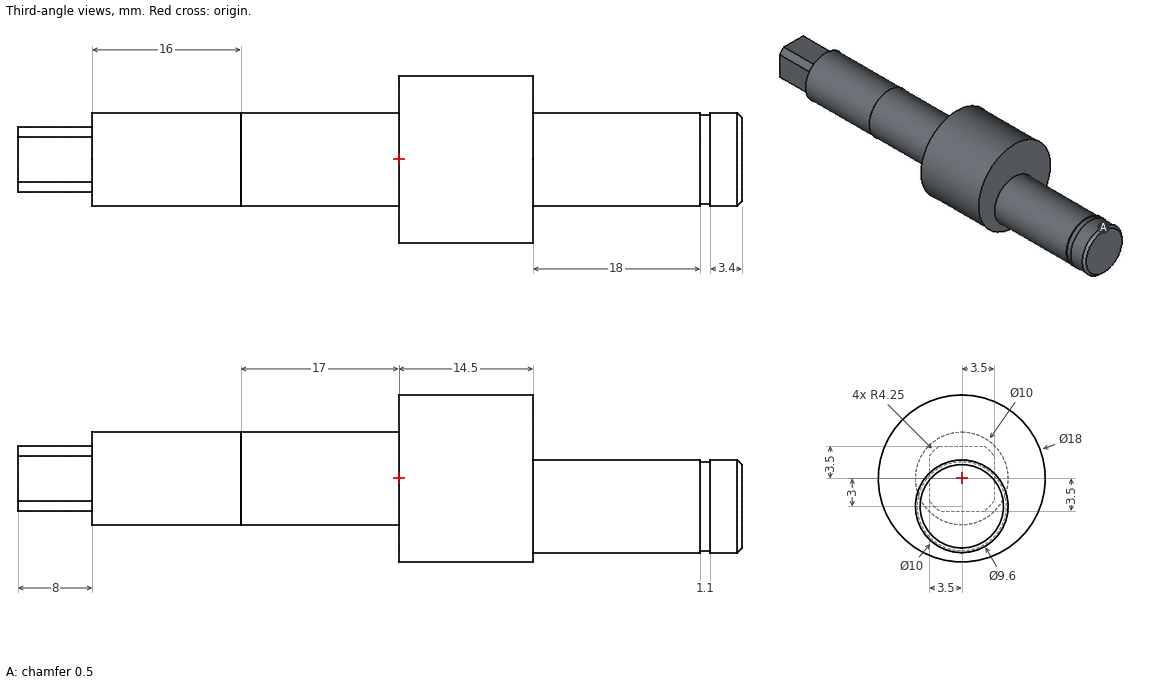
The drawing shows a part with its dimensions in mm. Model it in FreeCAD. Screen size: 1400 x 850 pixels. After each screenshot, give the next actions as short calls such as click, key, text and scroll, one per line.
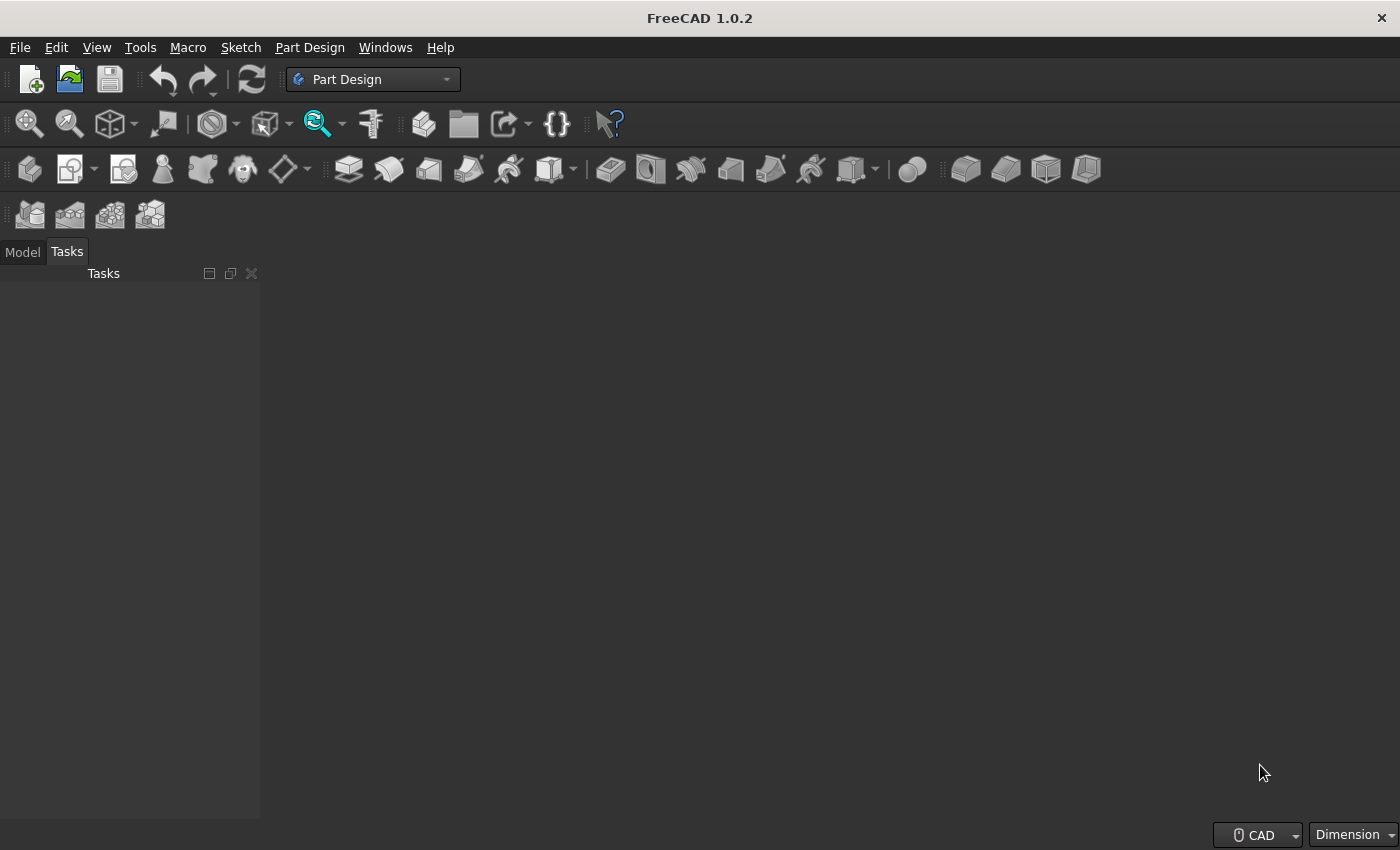
click(30, 80)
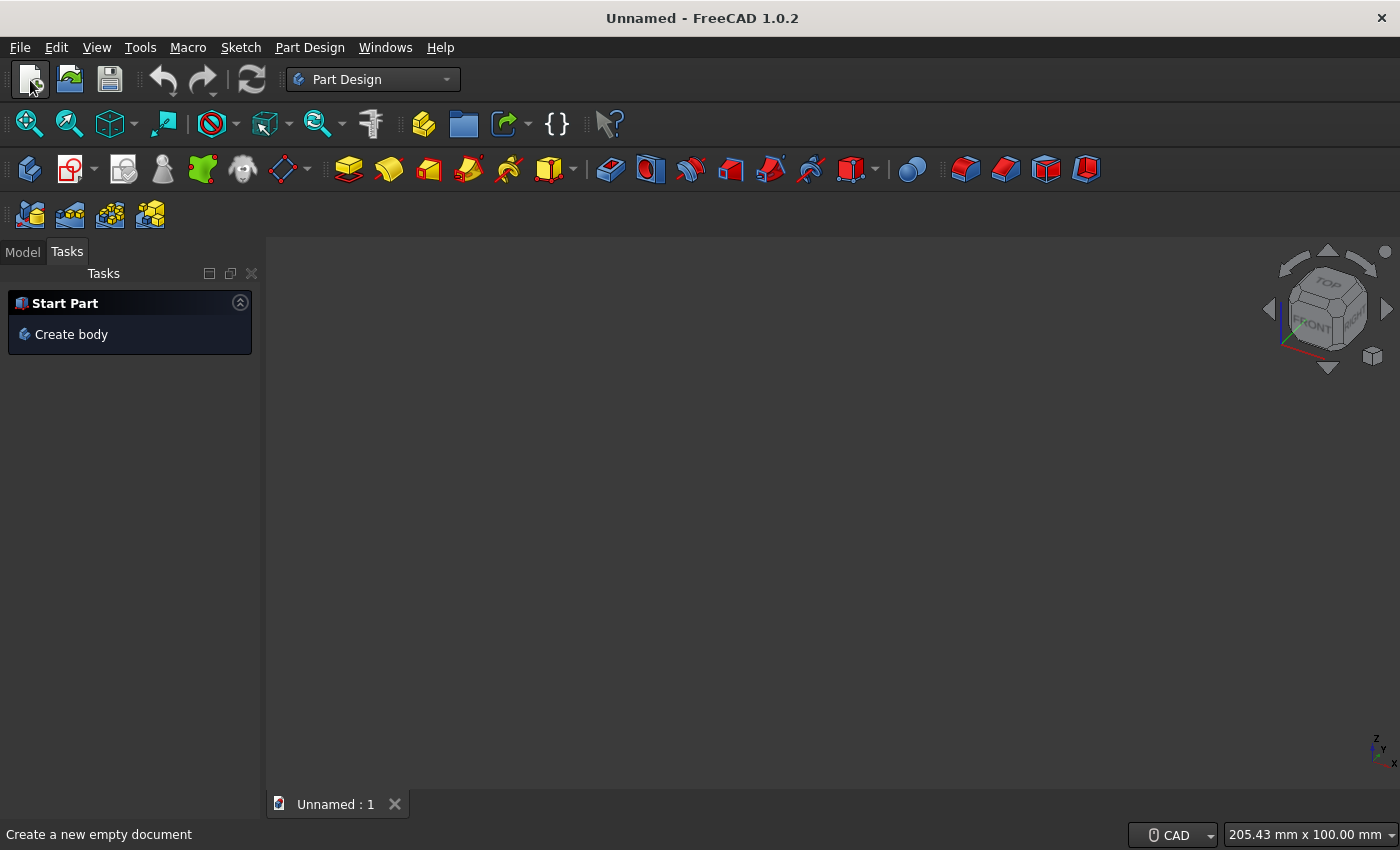
click(70, 170)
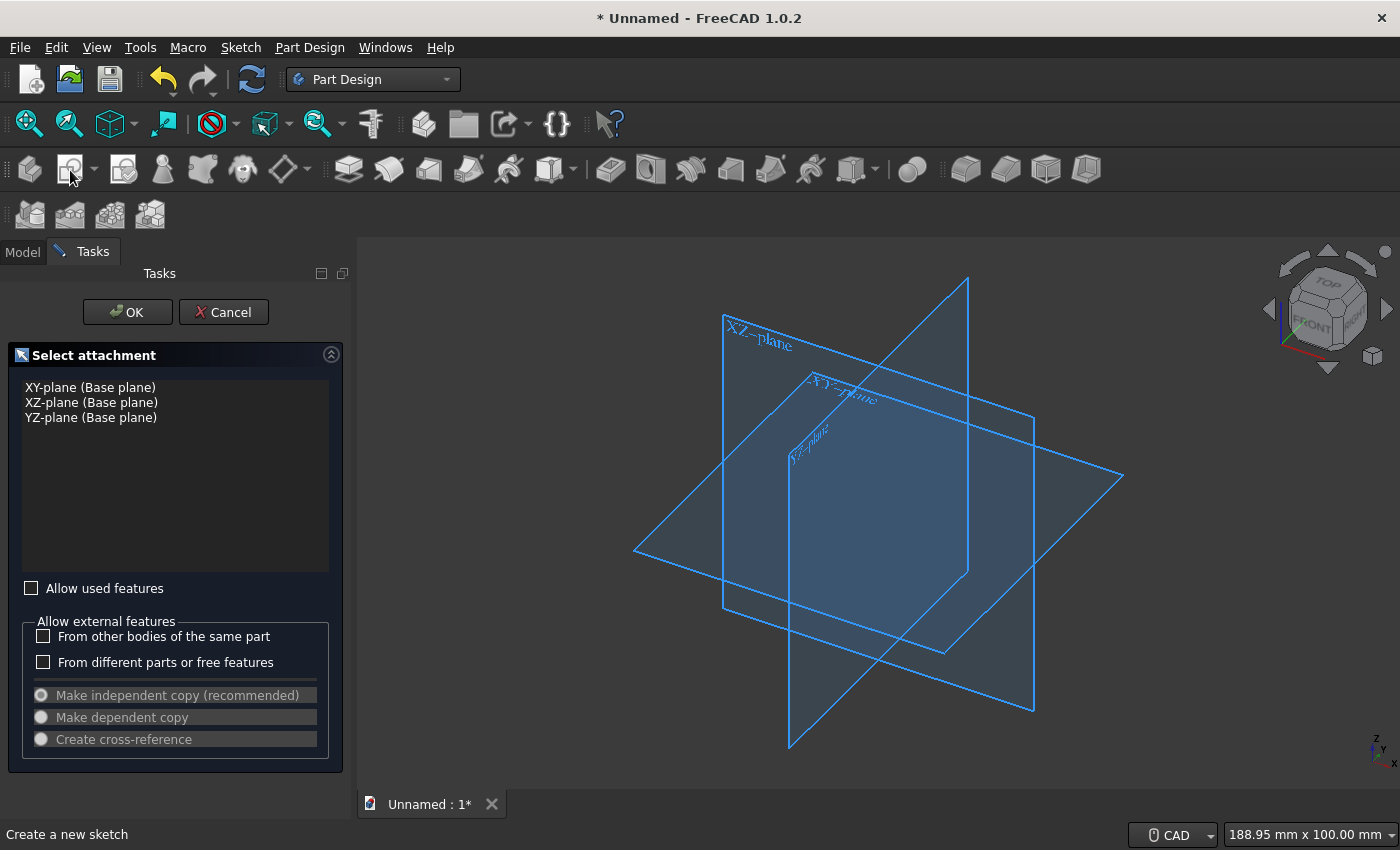
click(82, 418)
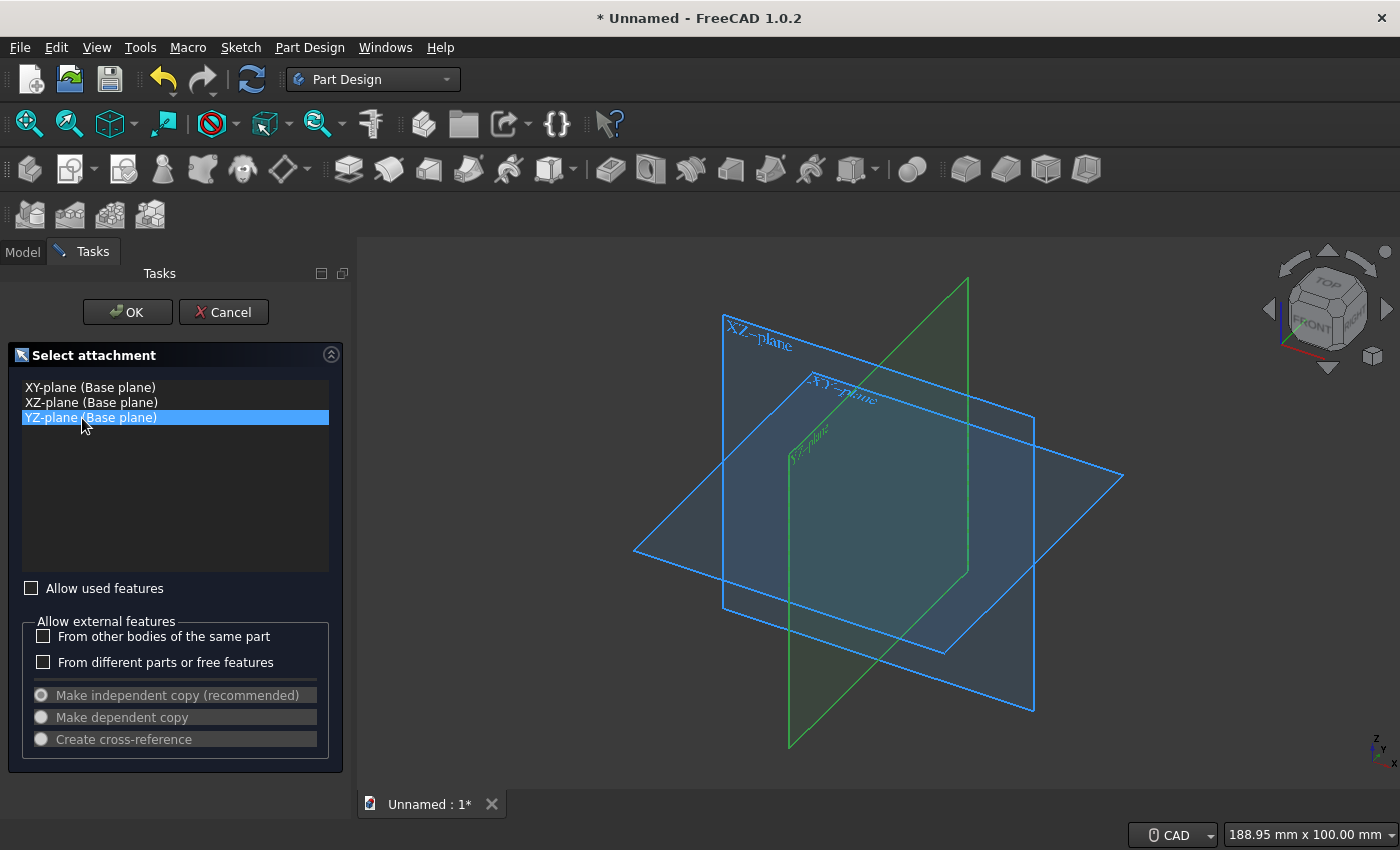
click(128, 312)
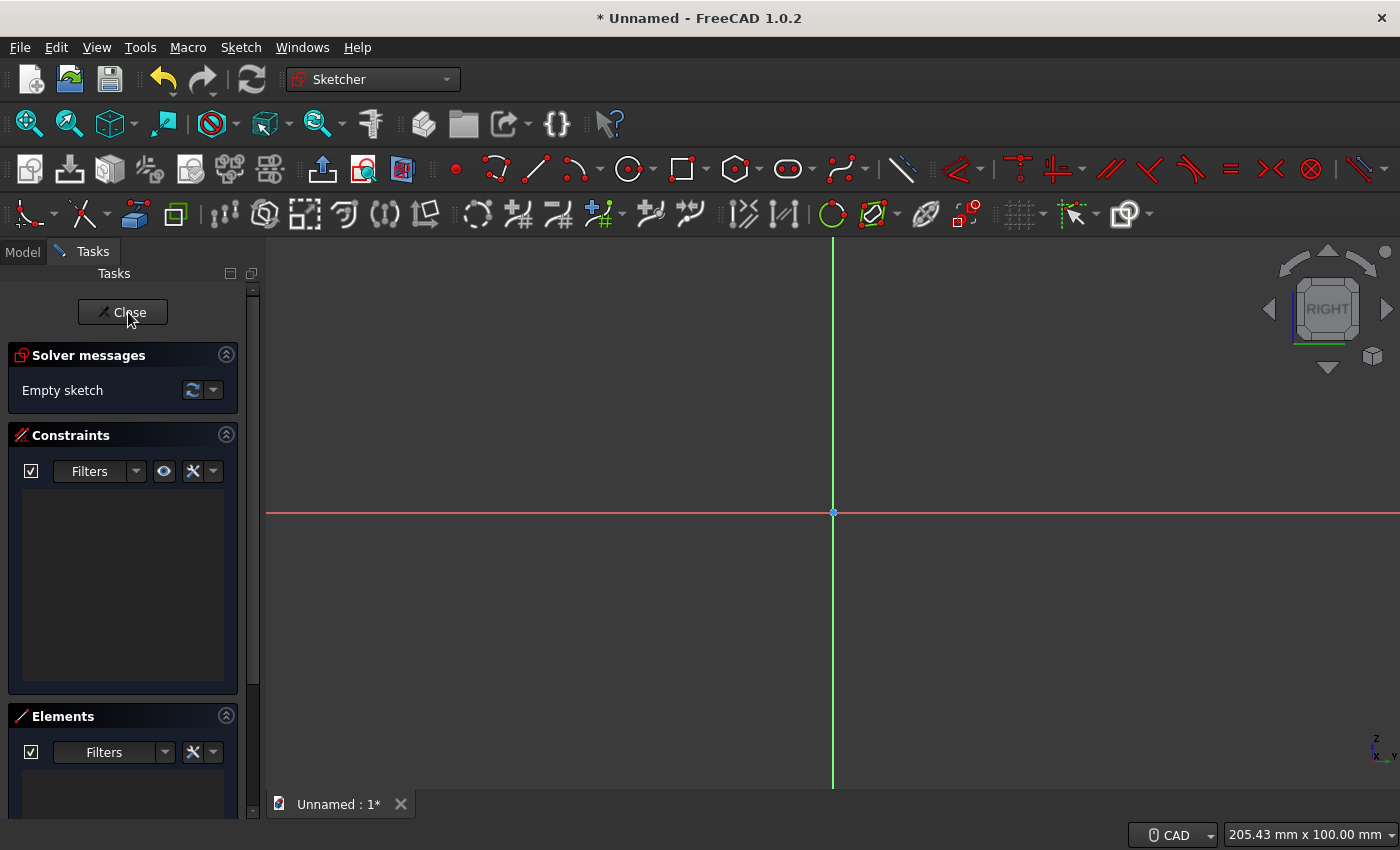
scroll(863, 513, up, 6)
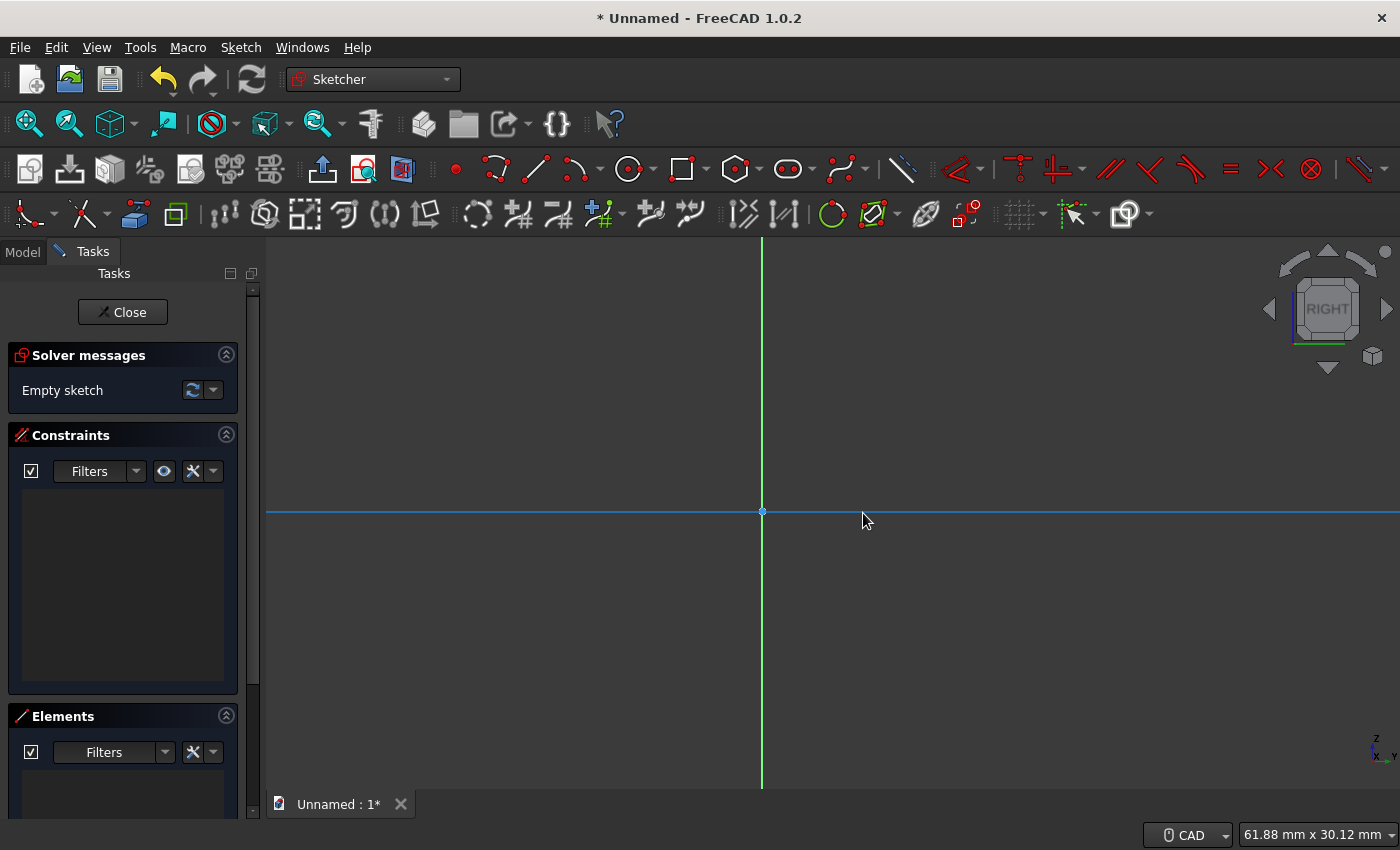
click(630, 170)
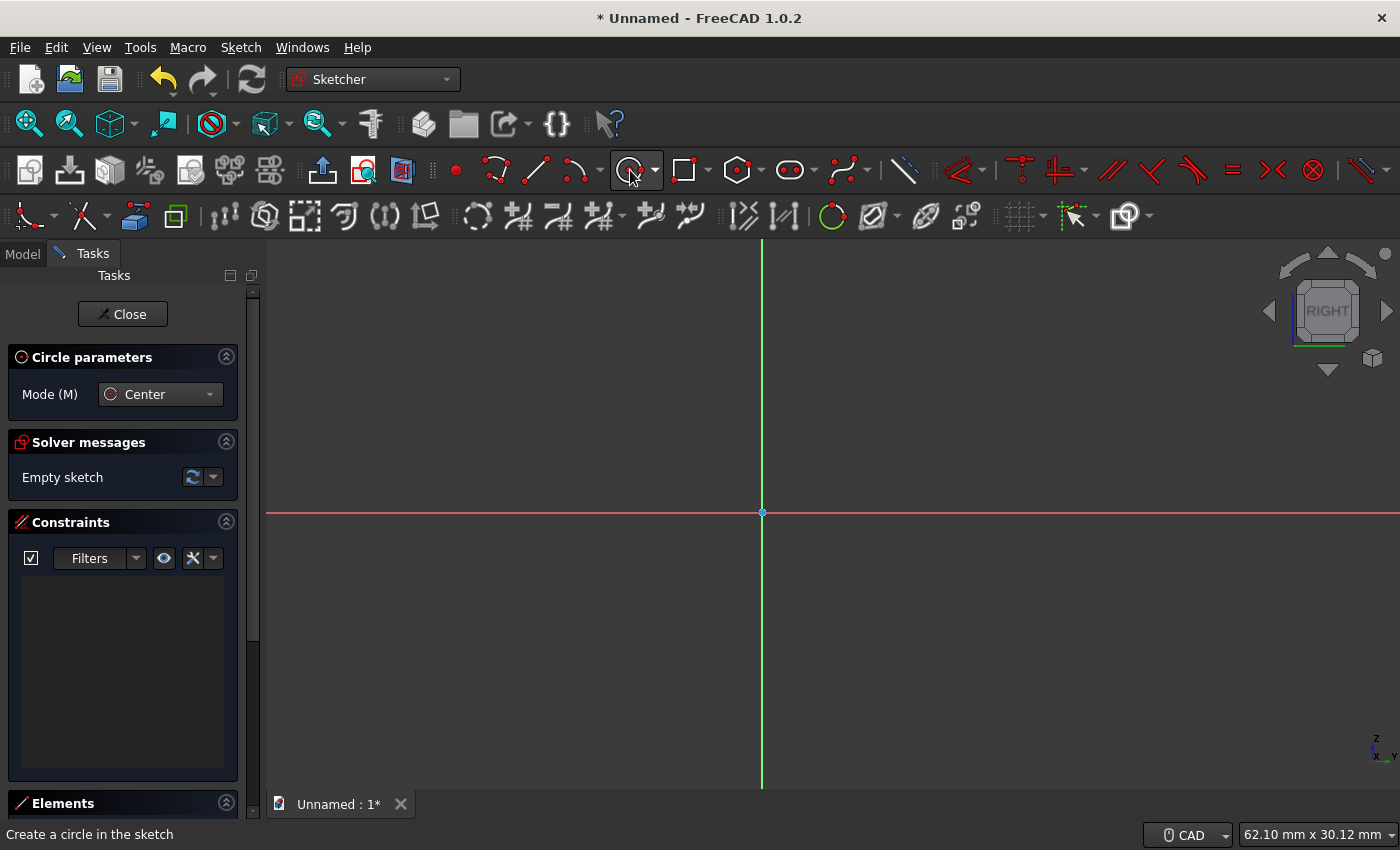
click(762, 513)
move(879, 397)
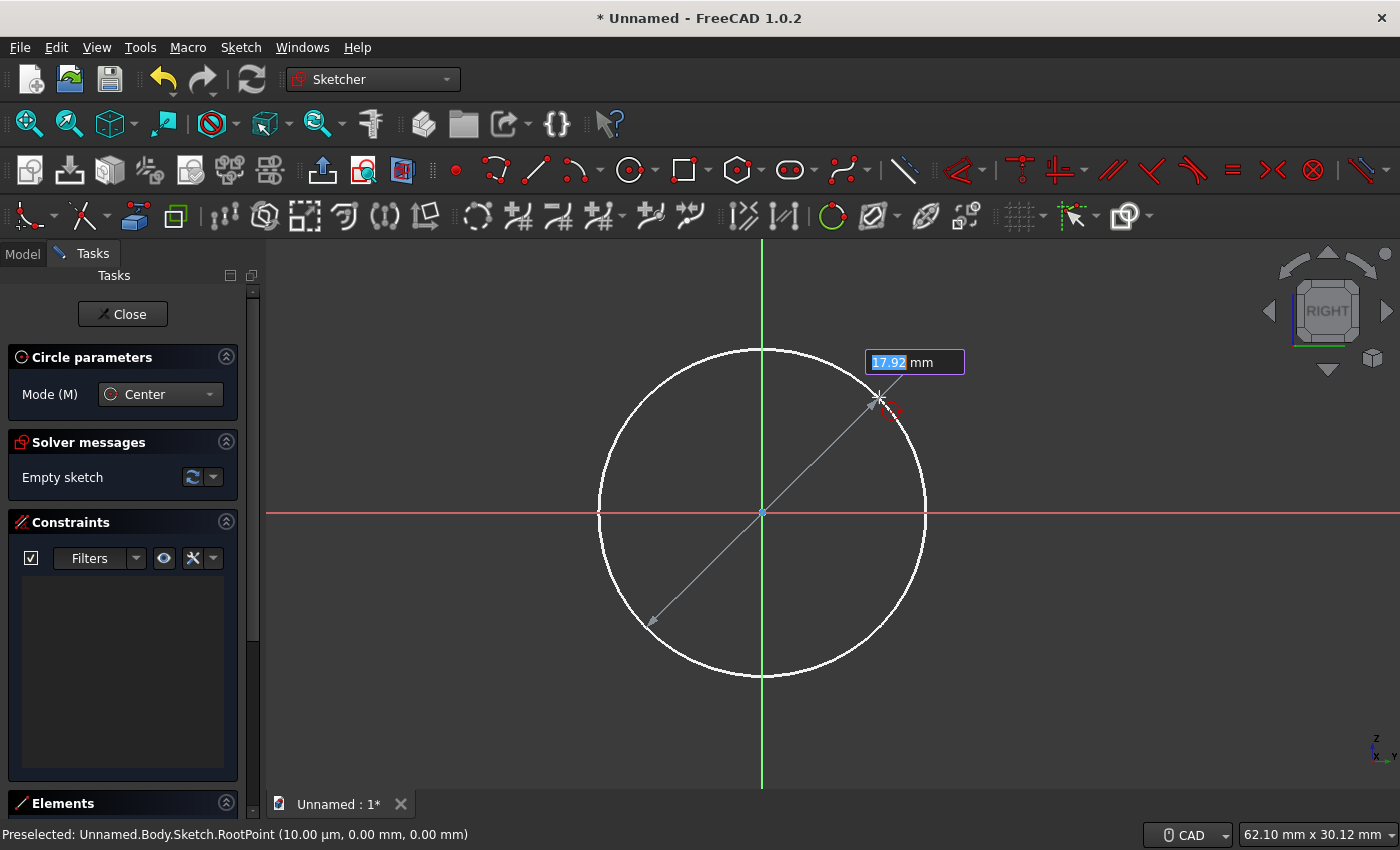
text(18)
key(Return)
key(Escape)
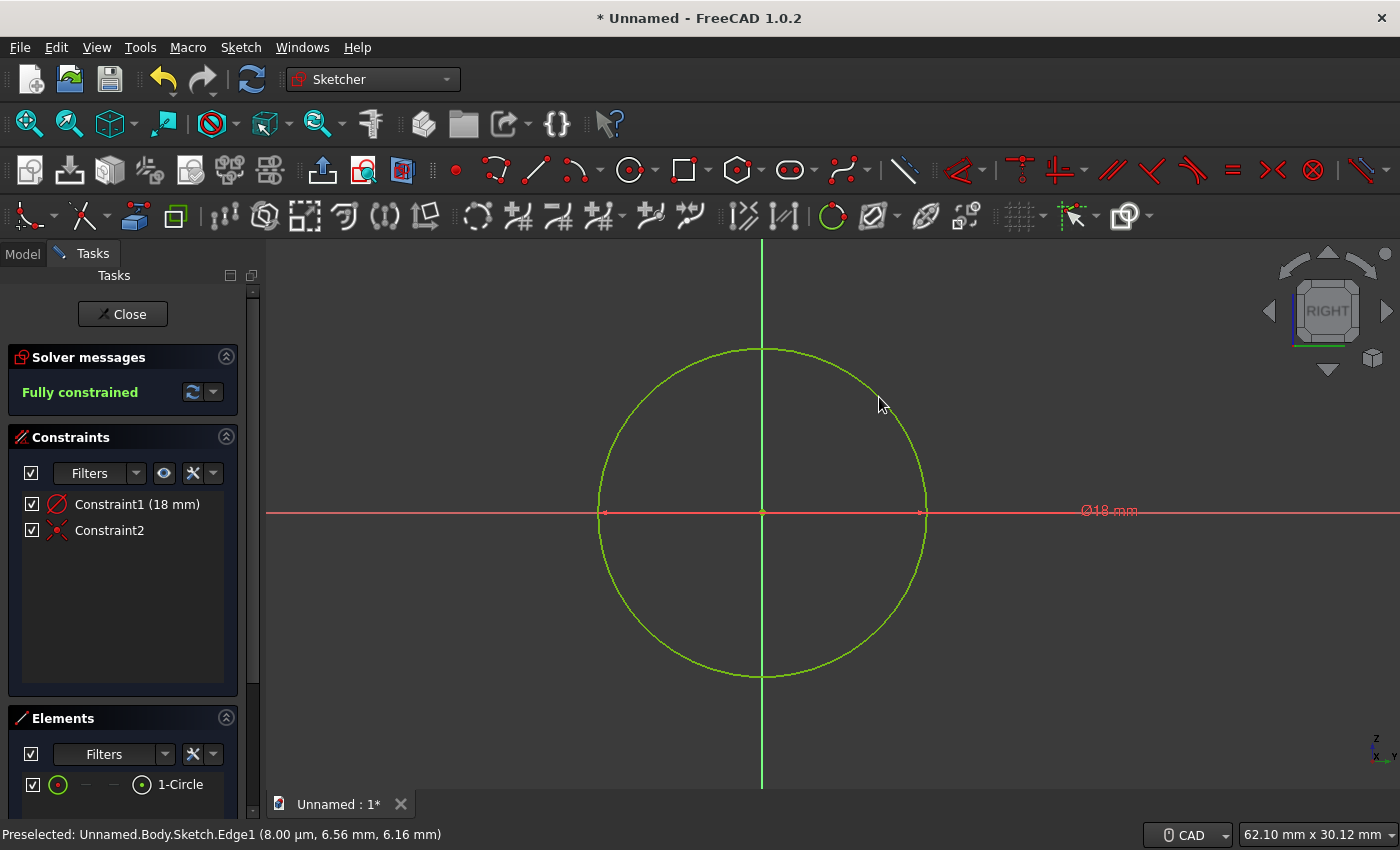
click(123, 314)